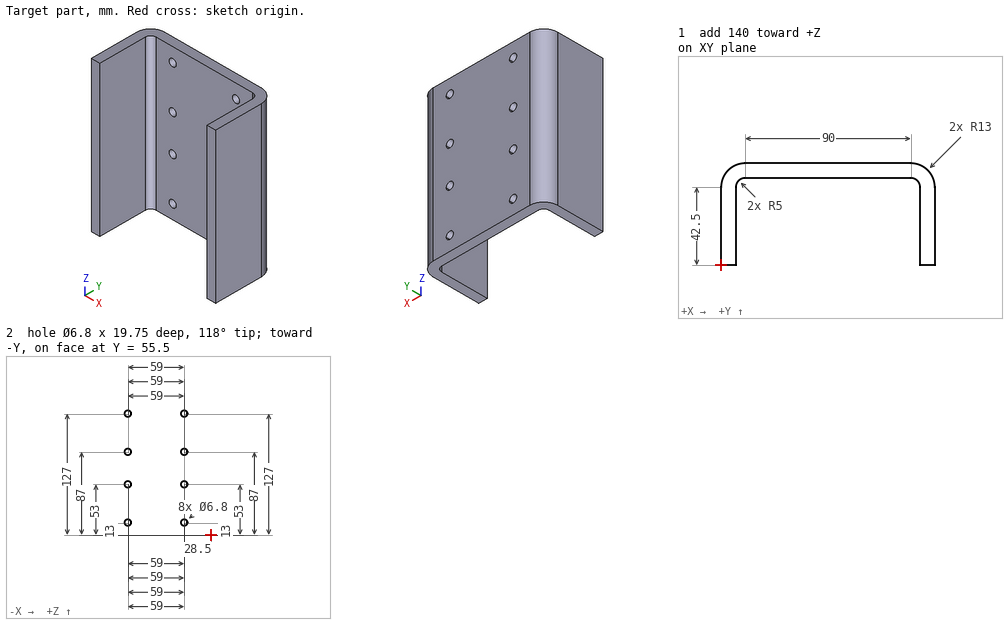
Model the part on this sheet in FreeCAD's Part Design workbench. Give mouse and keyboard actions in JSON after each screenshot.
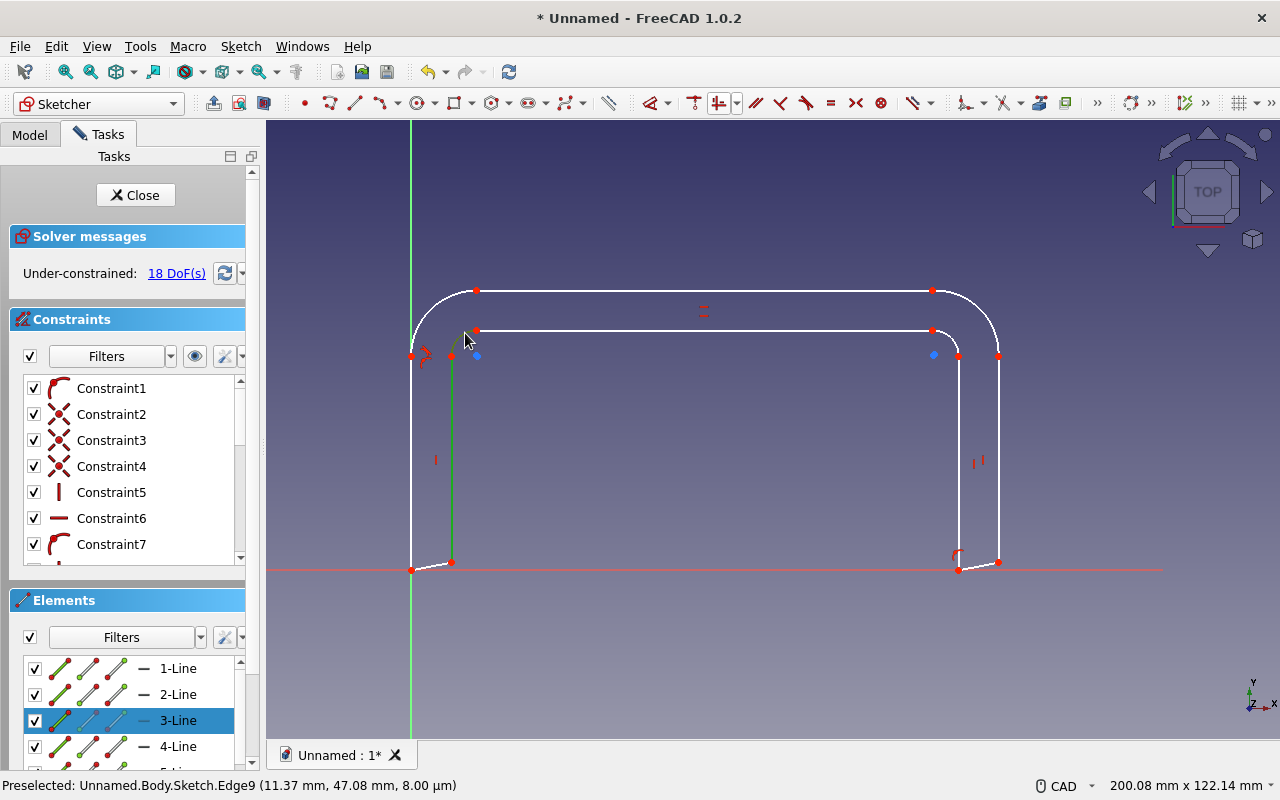
{"action": "key", "text": "t"}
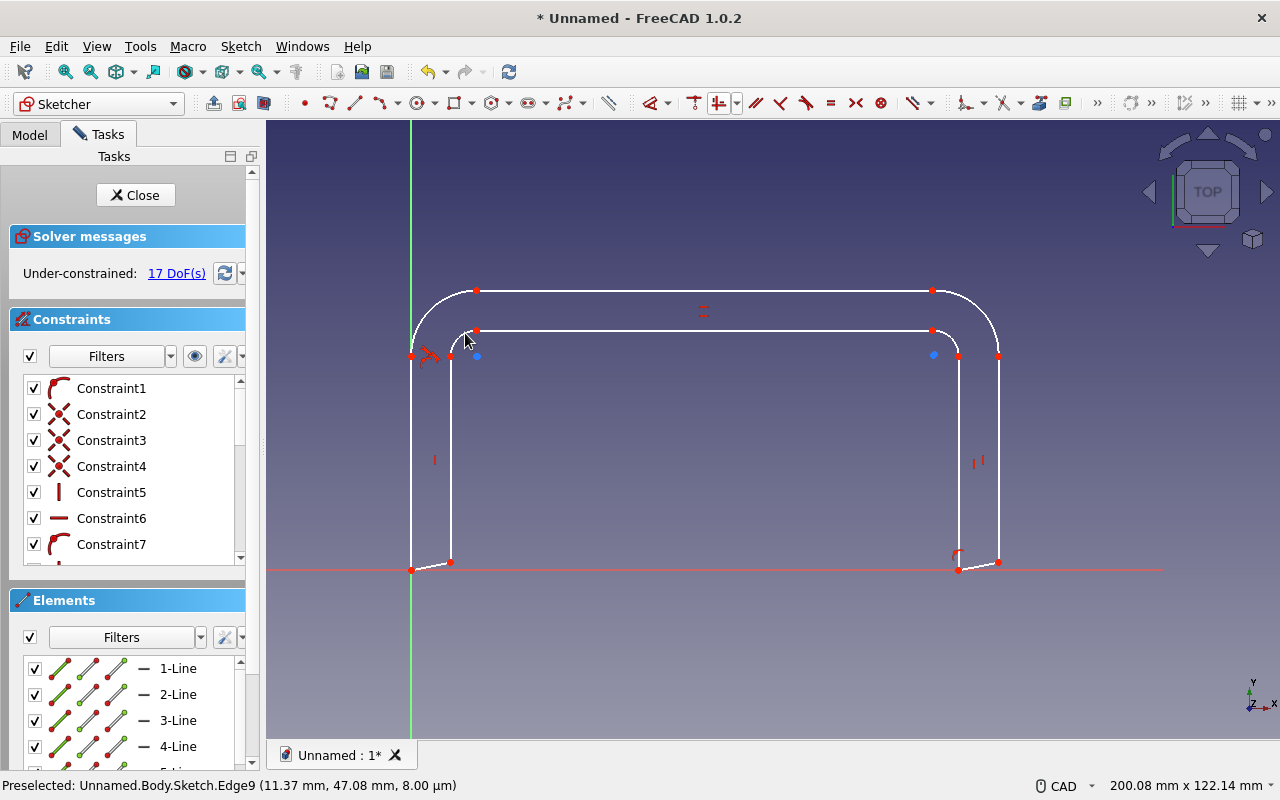
{"action": "left_click", "coordinate": [613, 331]}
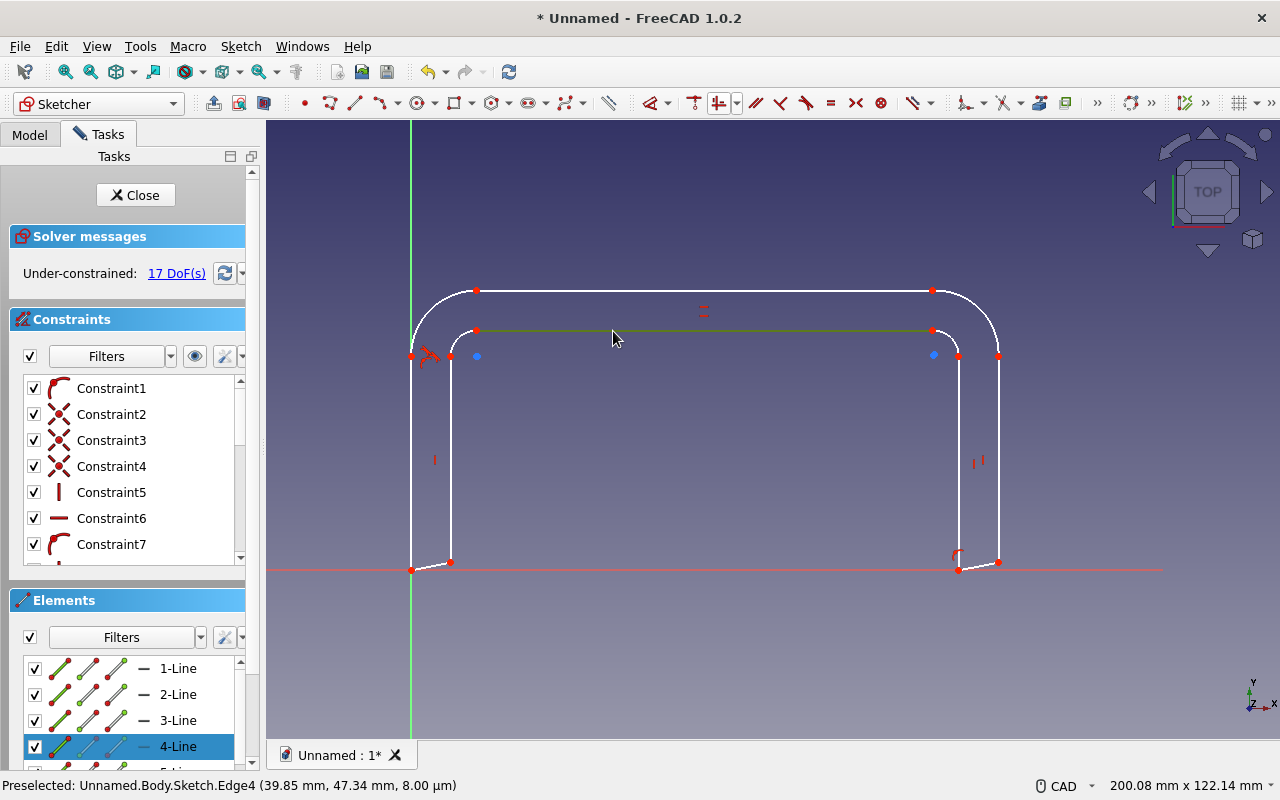
{"action": "left_click", "coordinate": [465, 333]}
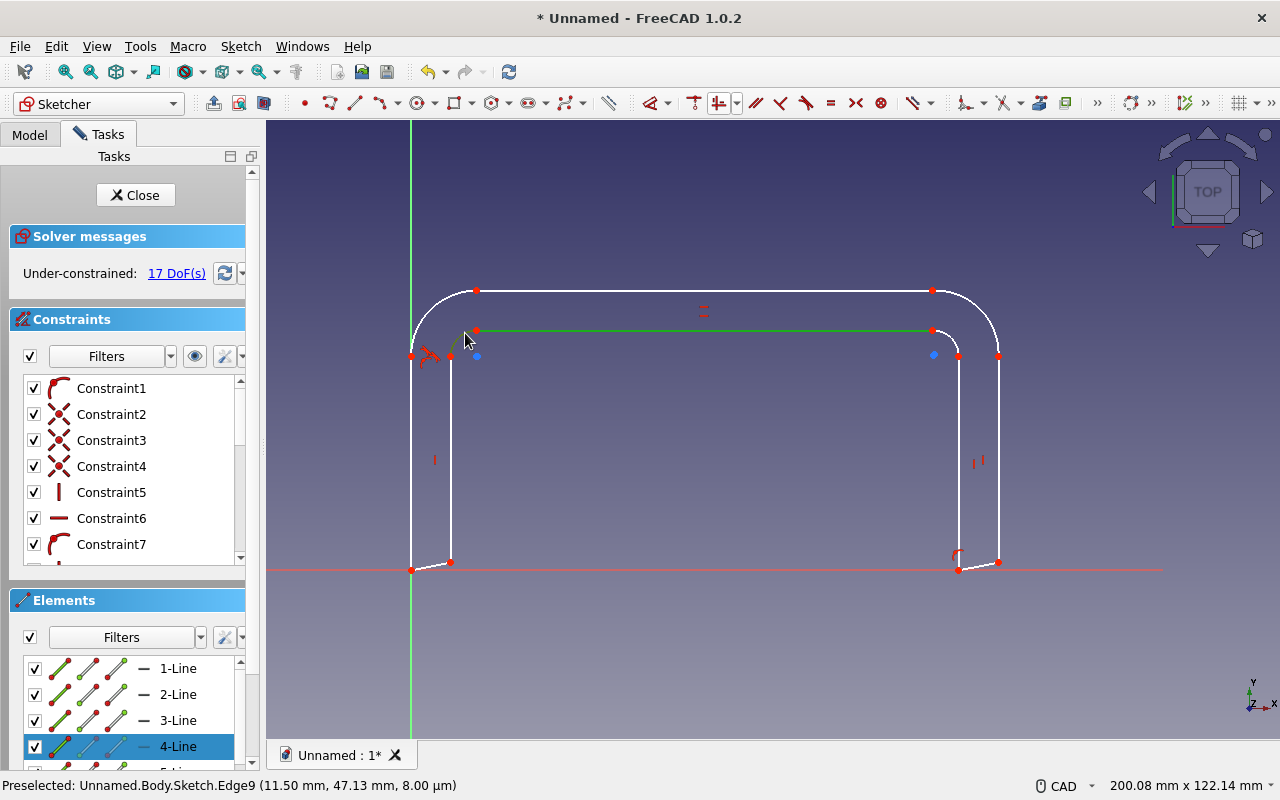
{"action": "key", "text": "t"}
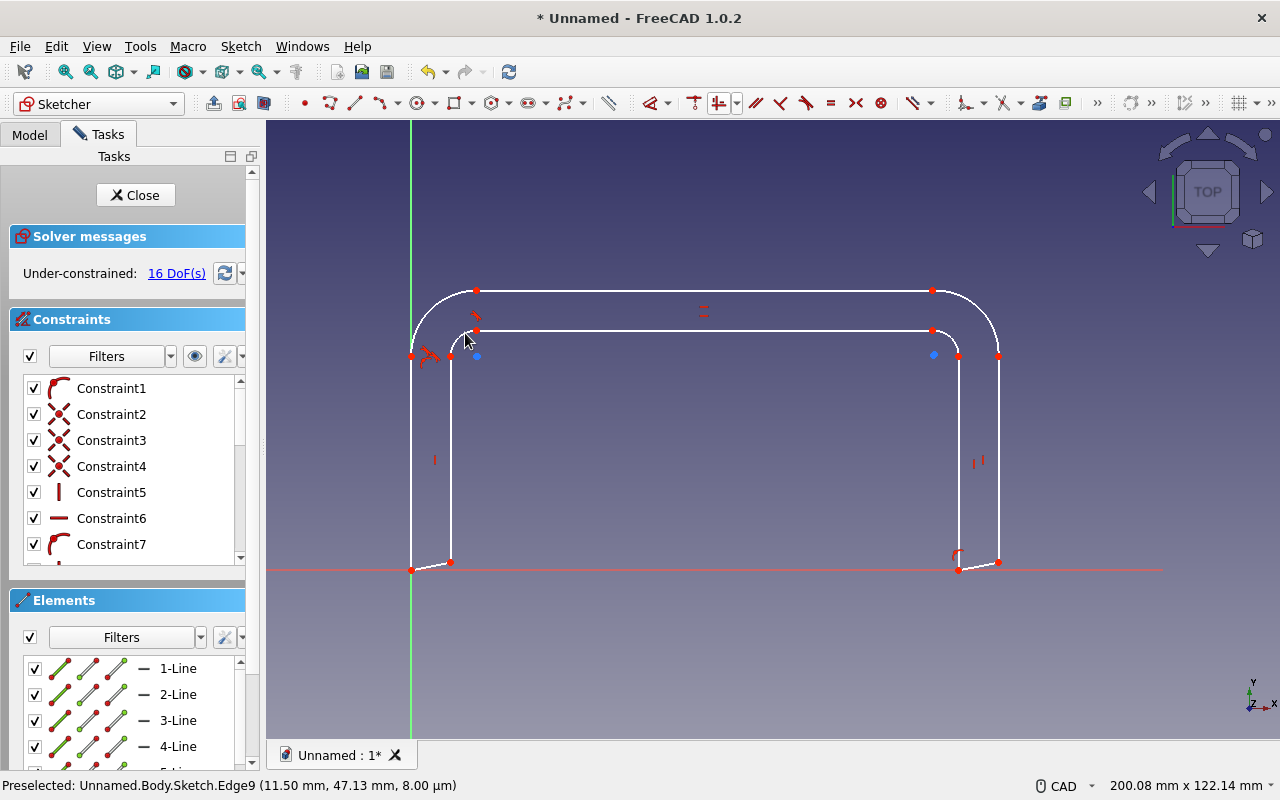
{"action": "left_click", "coordinate": [613, 331]}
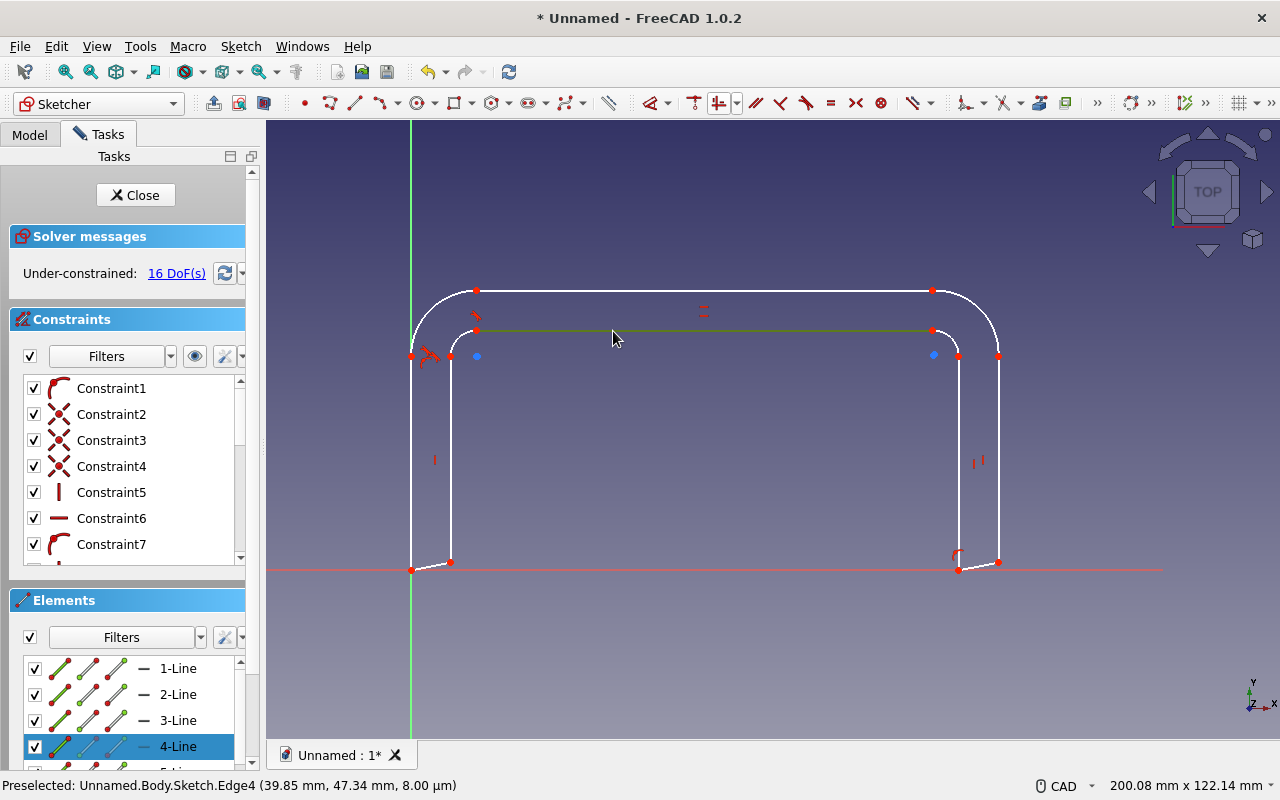
{"action": "left_click", "coordinate": [956, 345]}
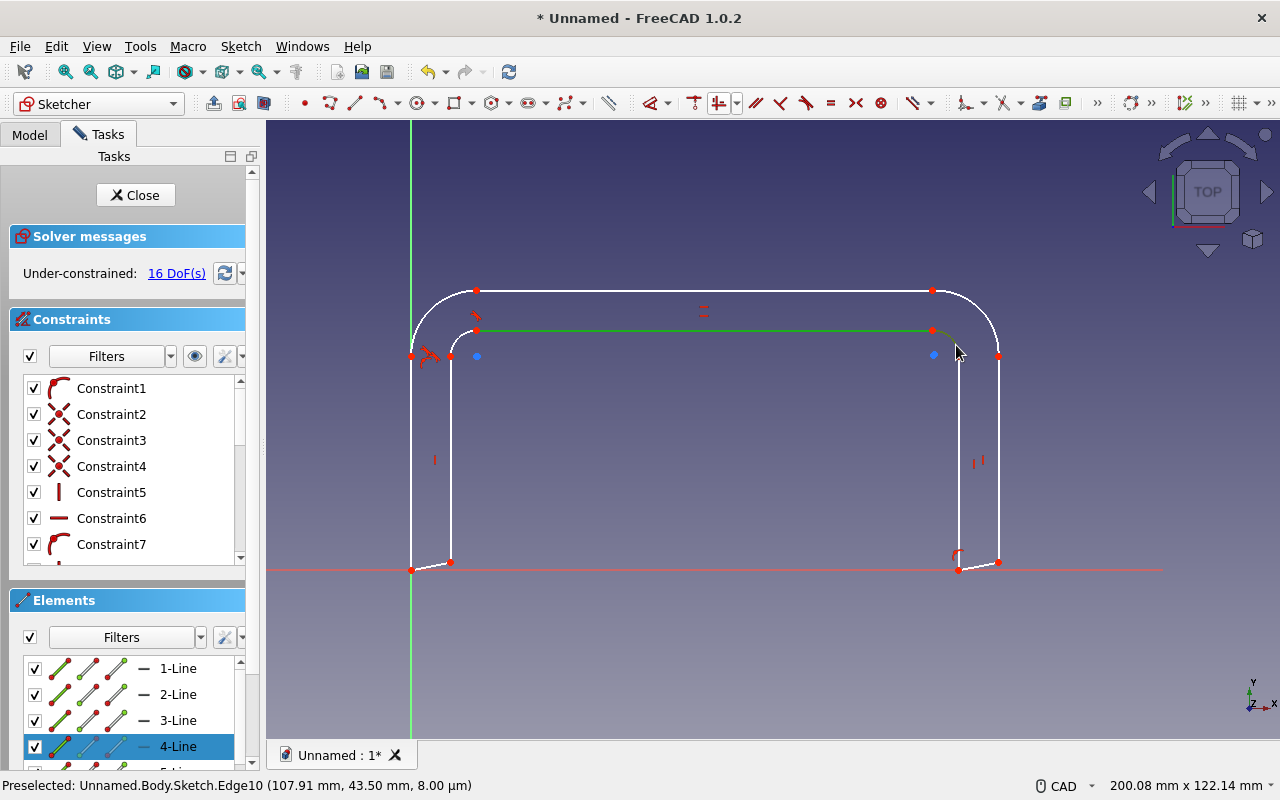
{"action": "left_click", "coordinate": [806, 104]}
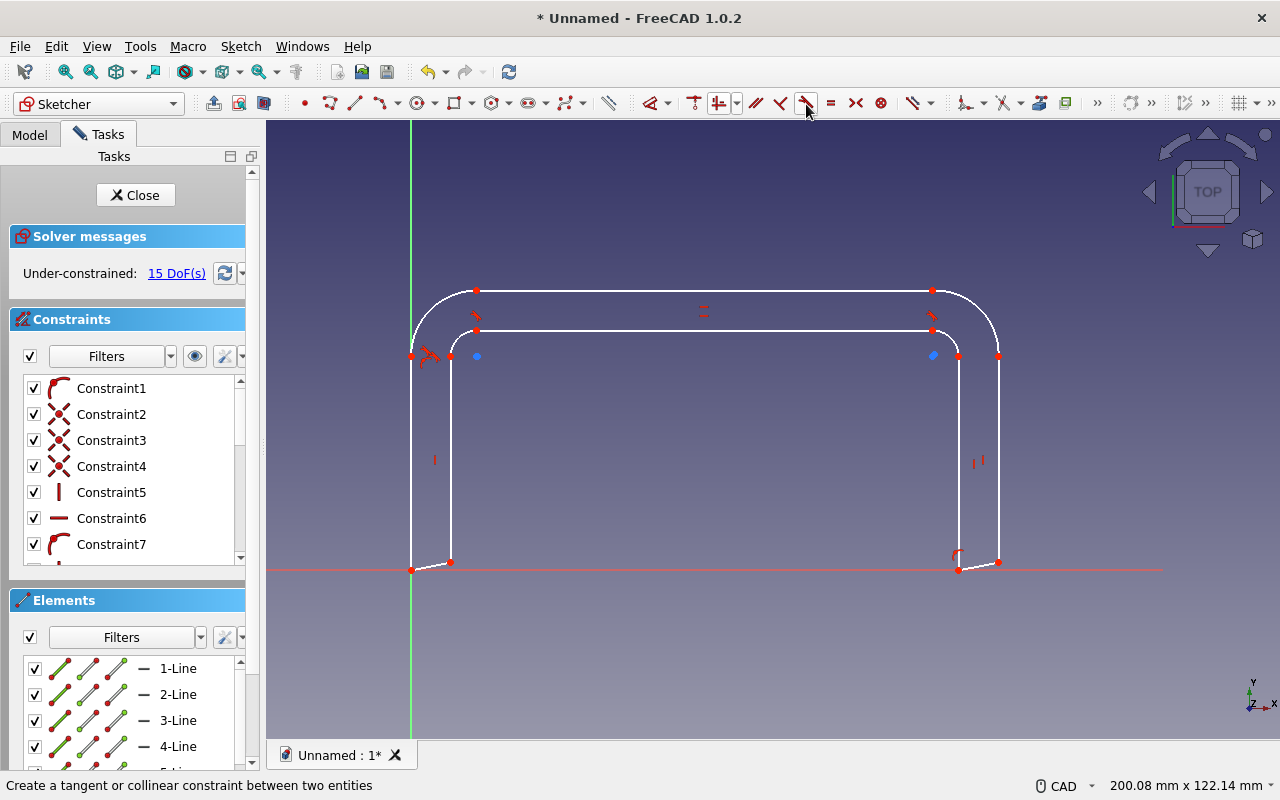
{"action": "left_click", "coordinate": [959, 421]}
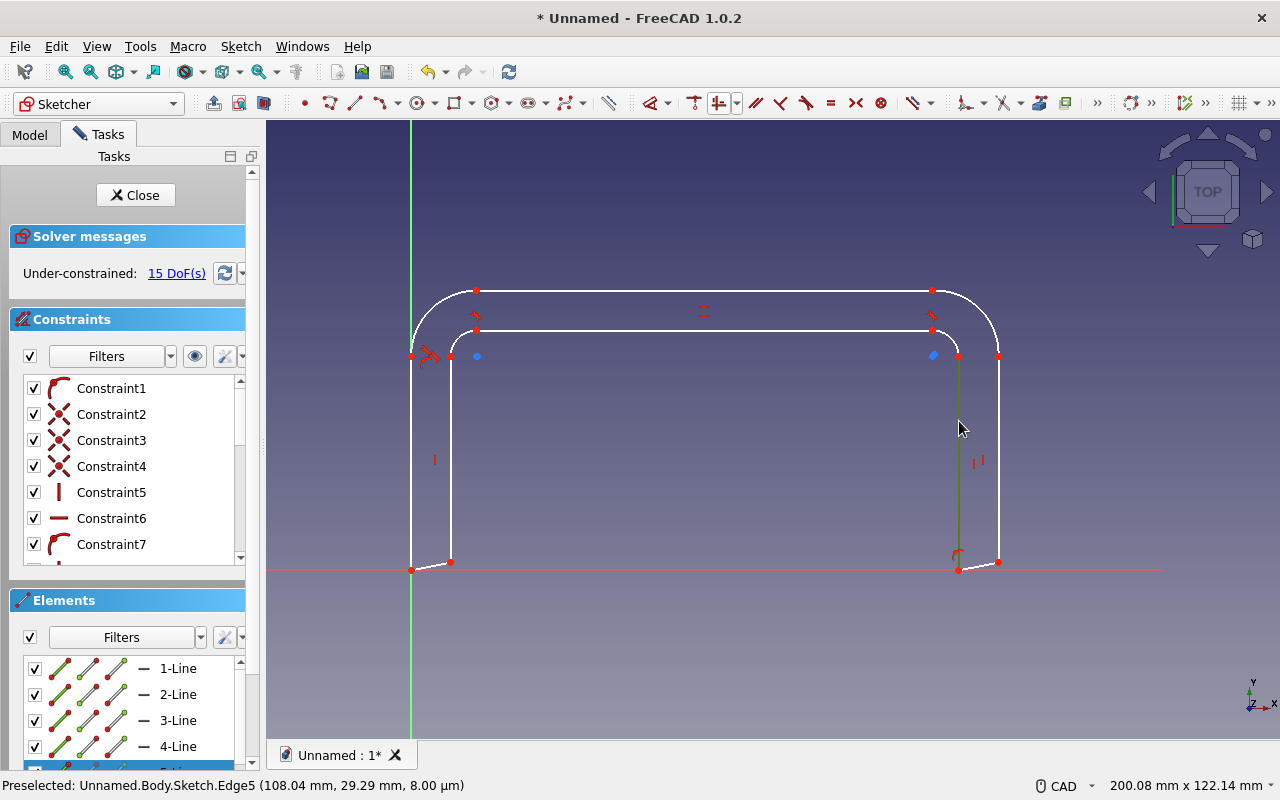
{"action": "left_click", "coordinate": [956, 345]}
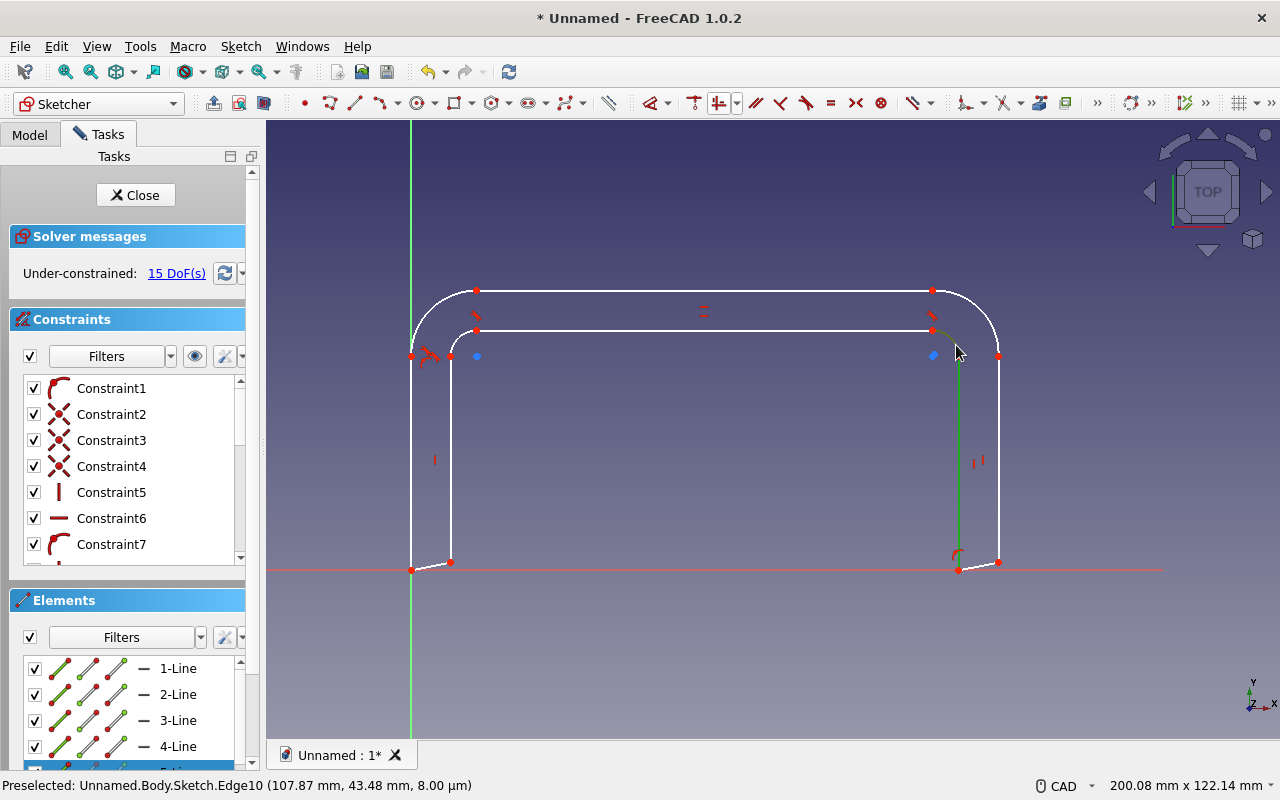
{"action": "left_click", "coordinate": [806, 104]}